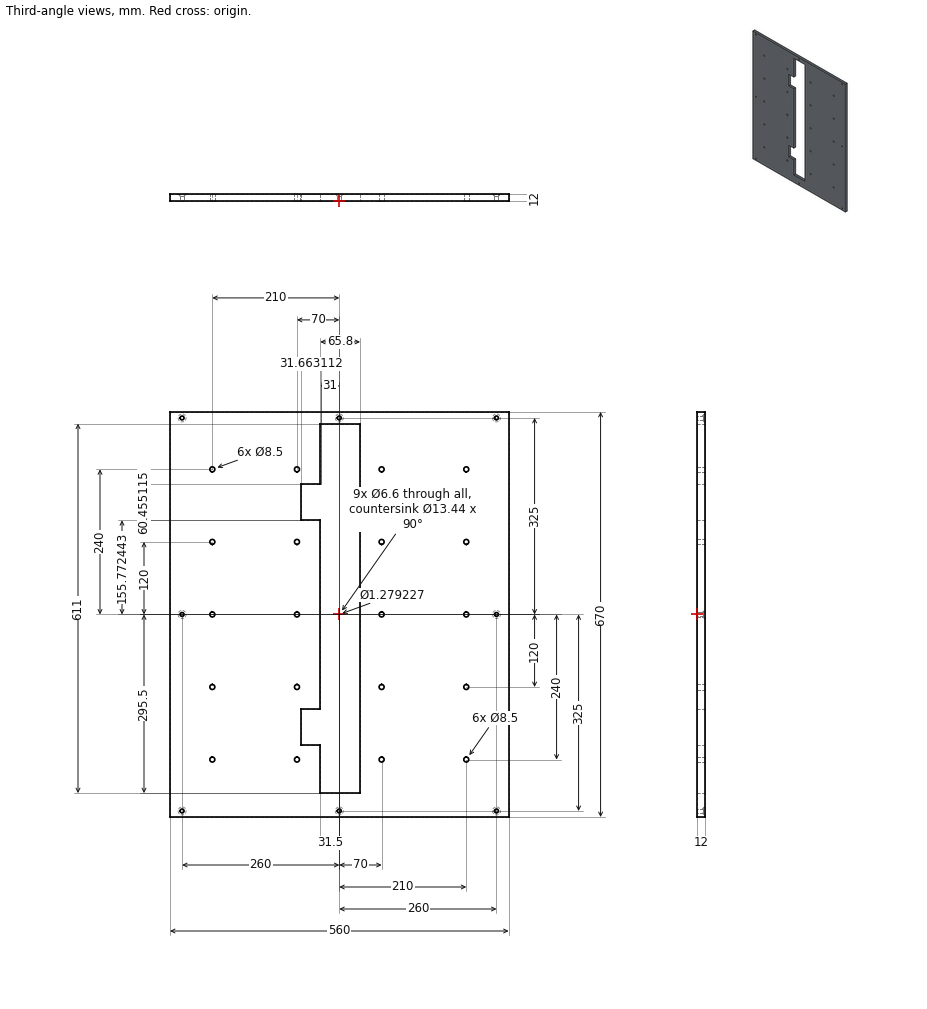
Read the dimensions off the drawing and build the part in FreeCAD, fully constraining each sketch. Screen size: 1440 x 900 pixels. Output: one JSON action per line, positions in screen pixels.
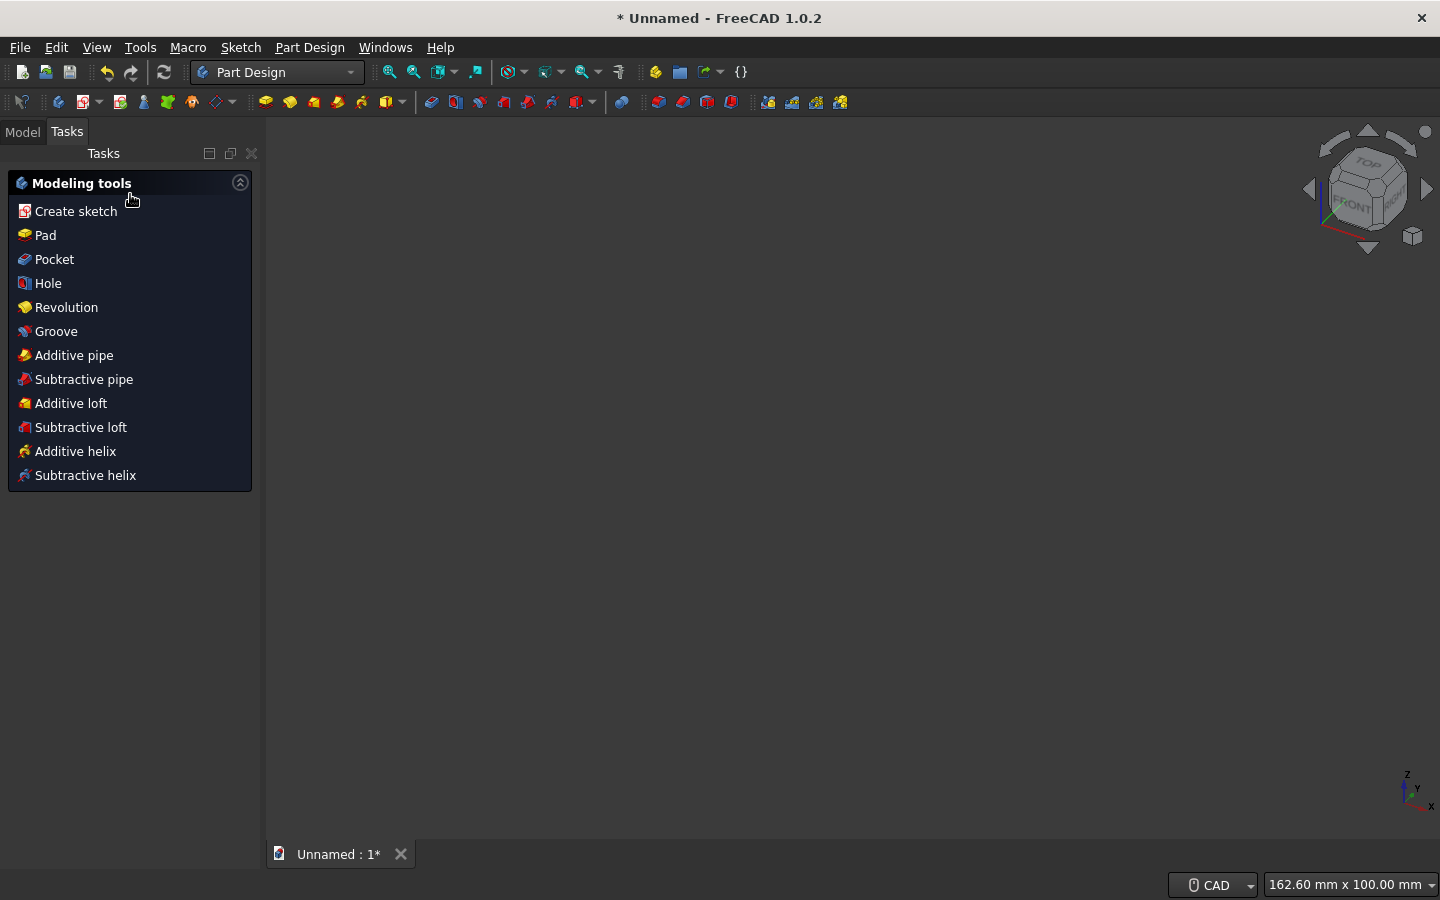
{"action": "left_click", "coordinate": [266, 102]}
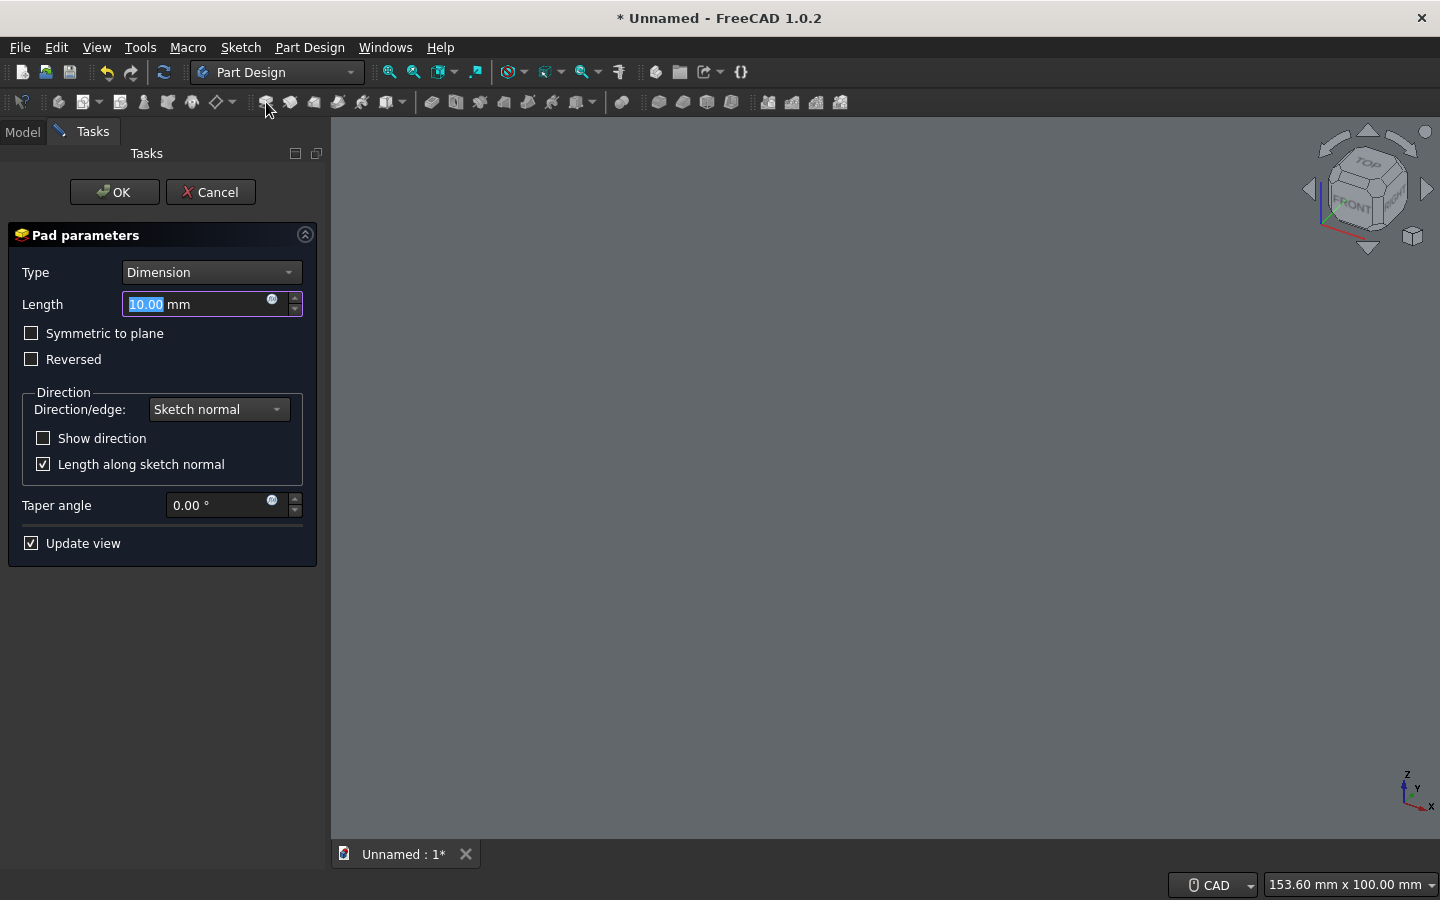
{"action": "type", "text": "12"}
{"action": "key", "text": "Tab"}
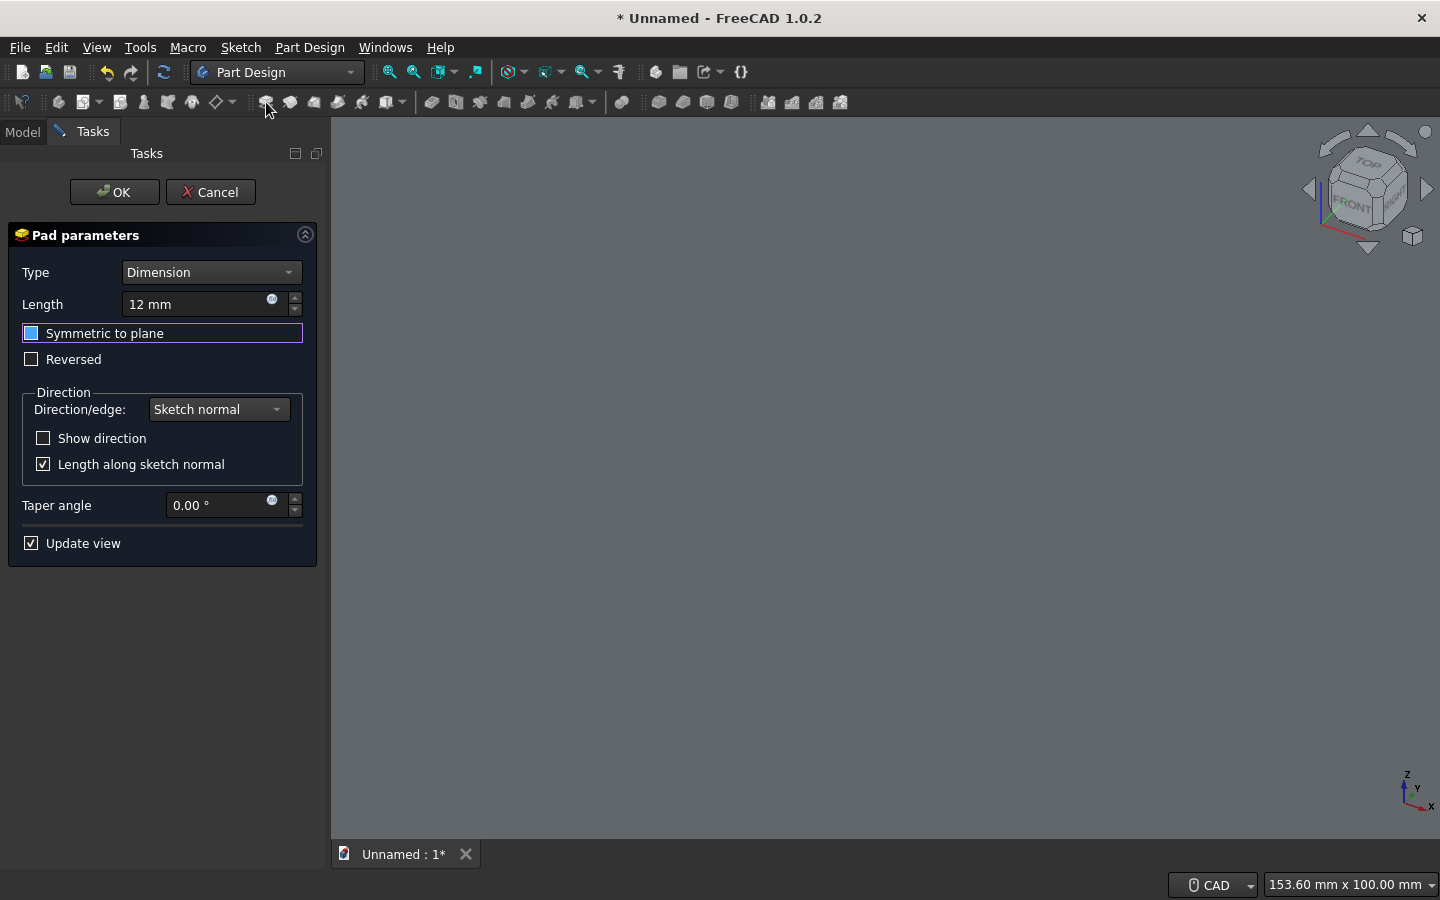
{"action": "left_click", "coordinate": [30, 359]}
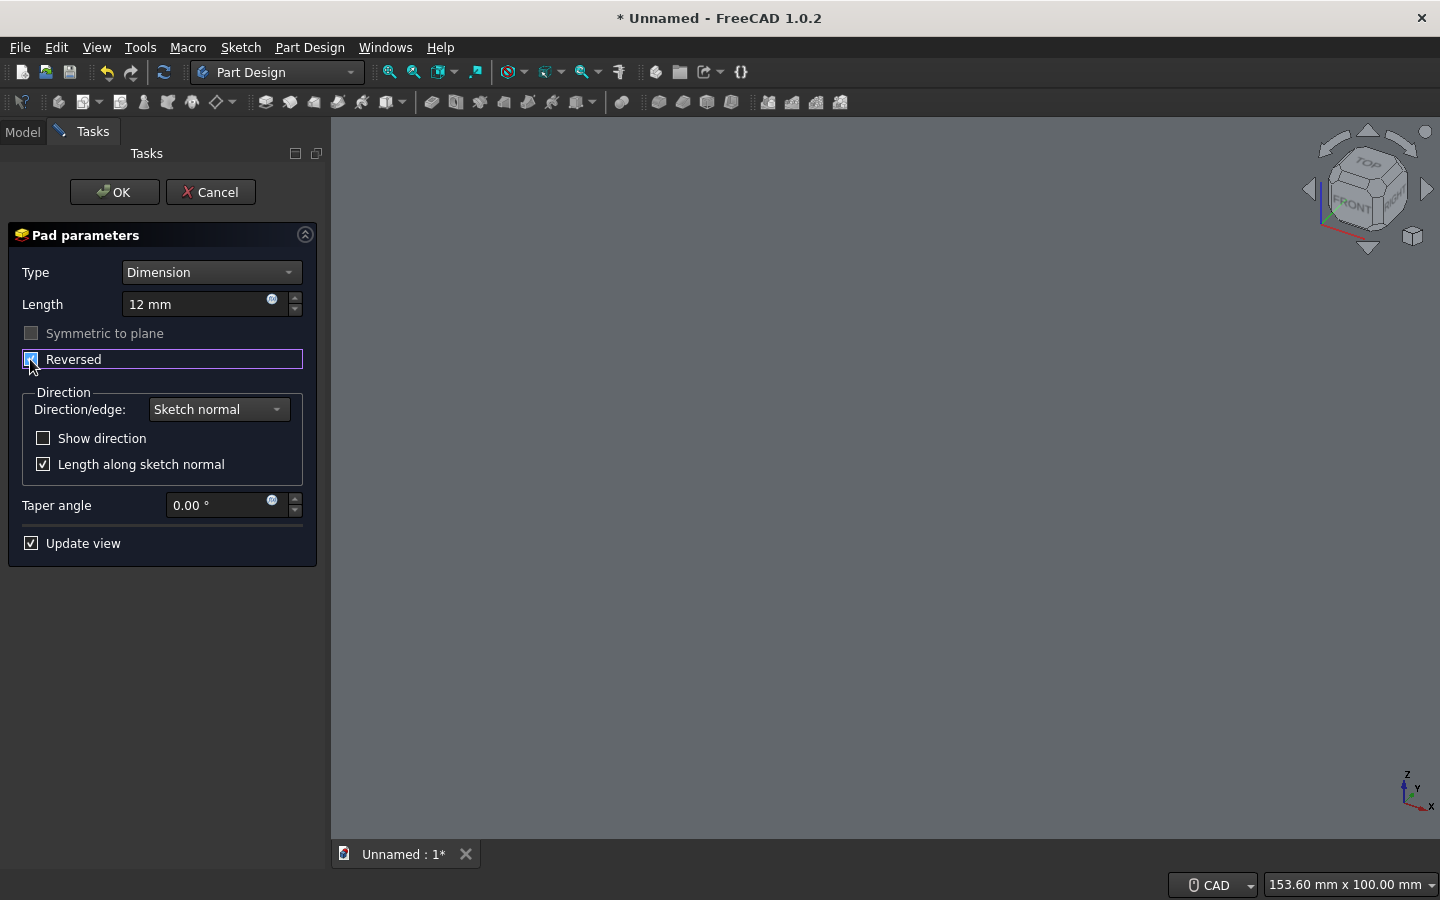
{"action": "left_click", "coordinate": [115, 192]}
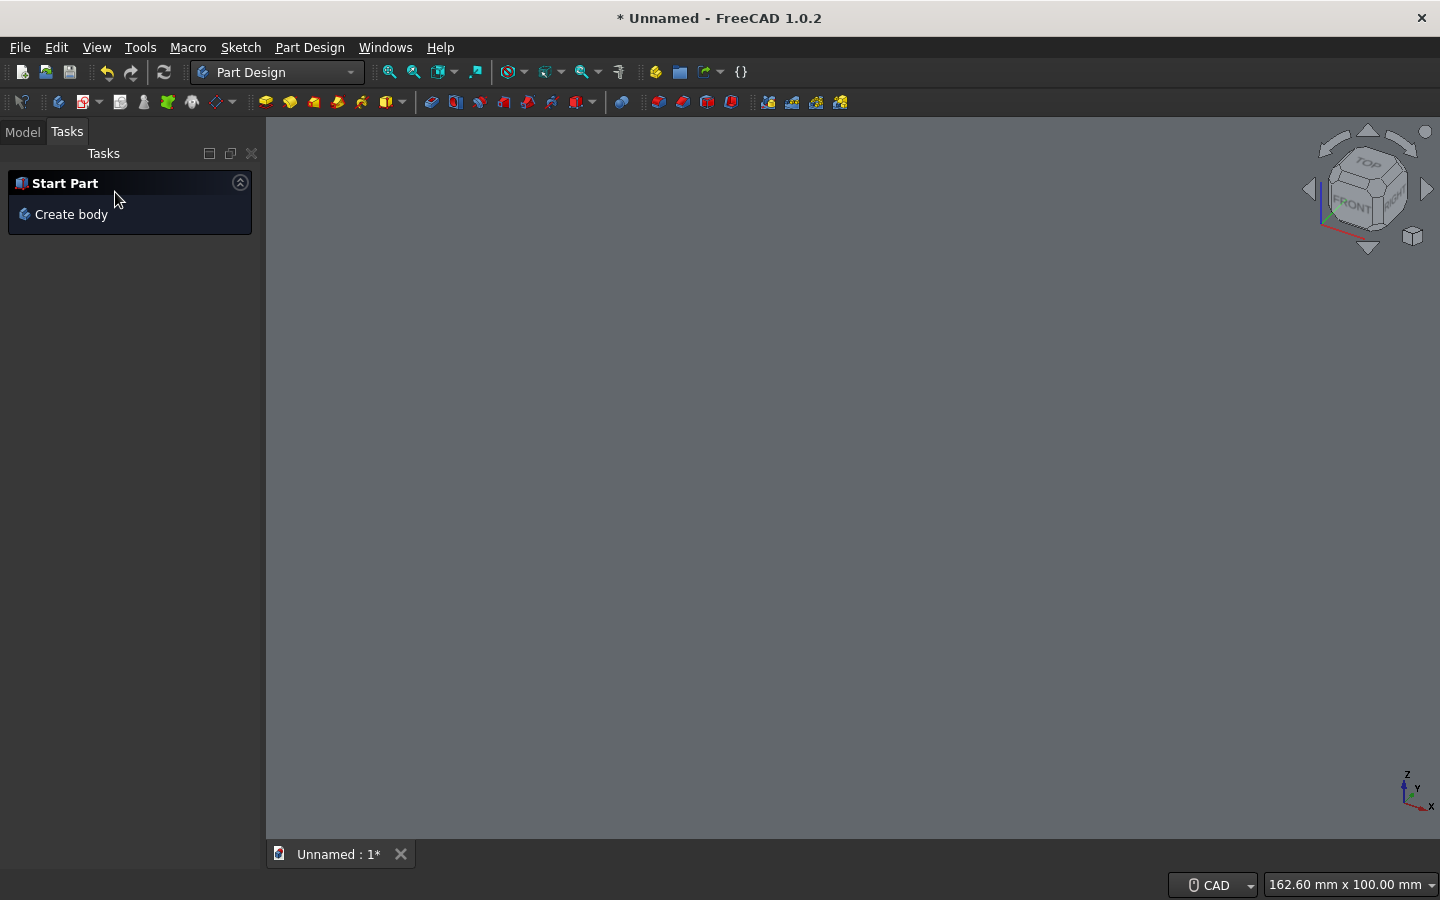
{"action": "left_click", "coordinate": [390, 72]}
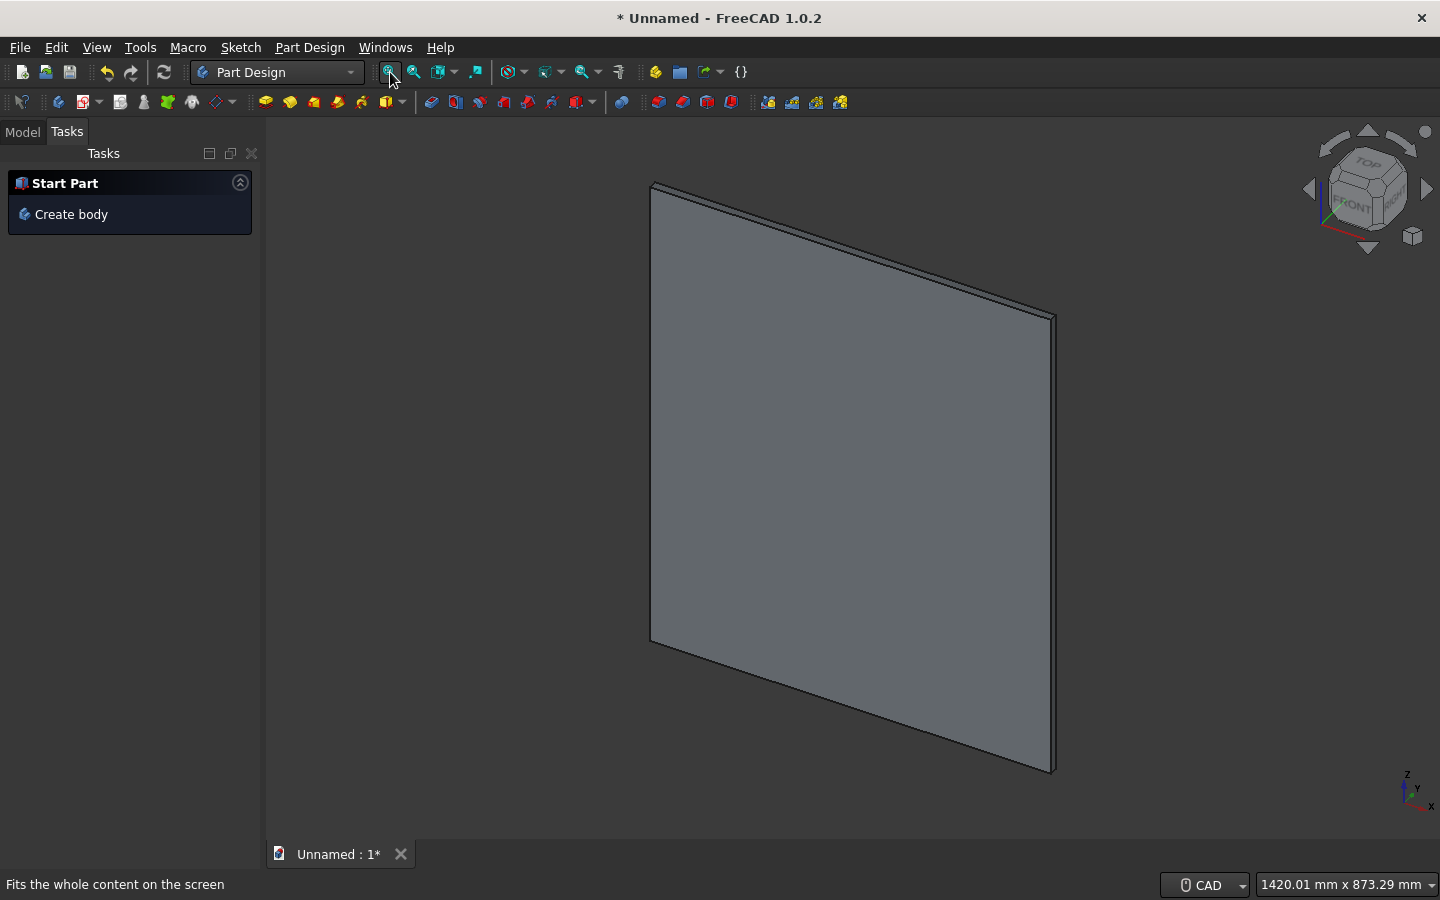
{"action": "key", "text": "4"}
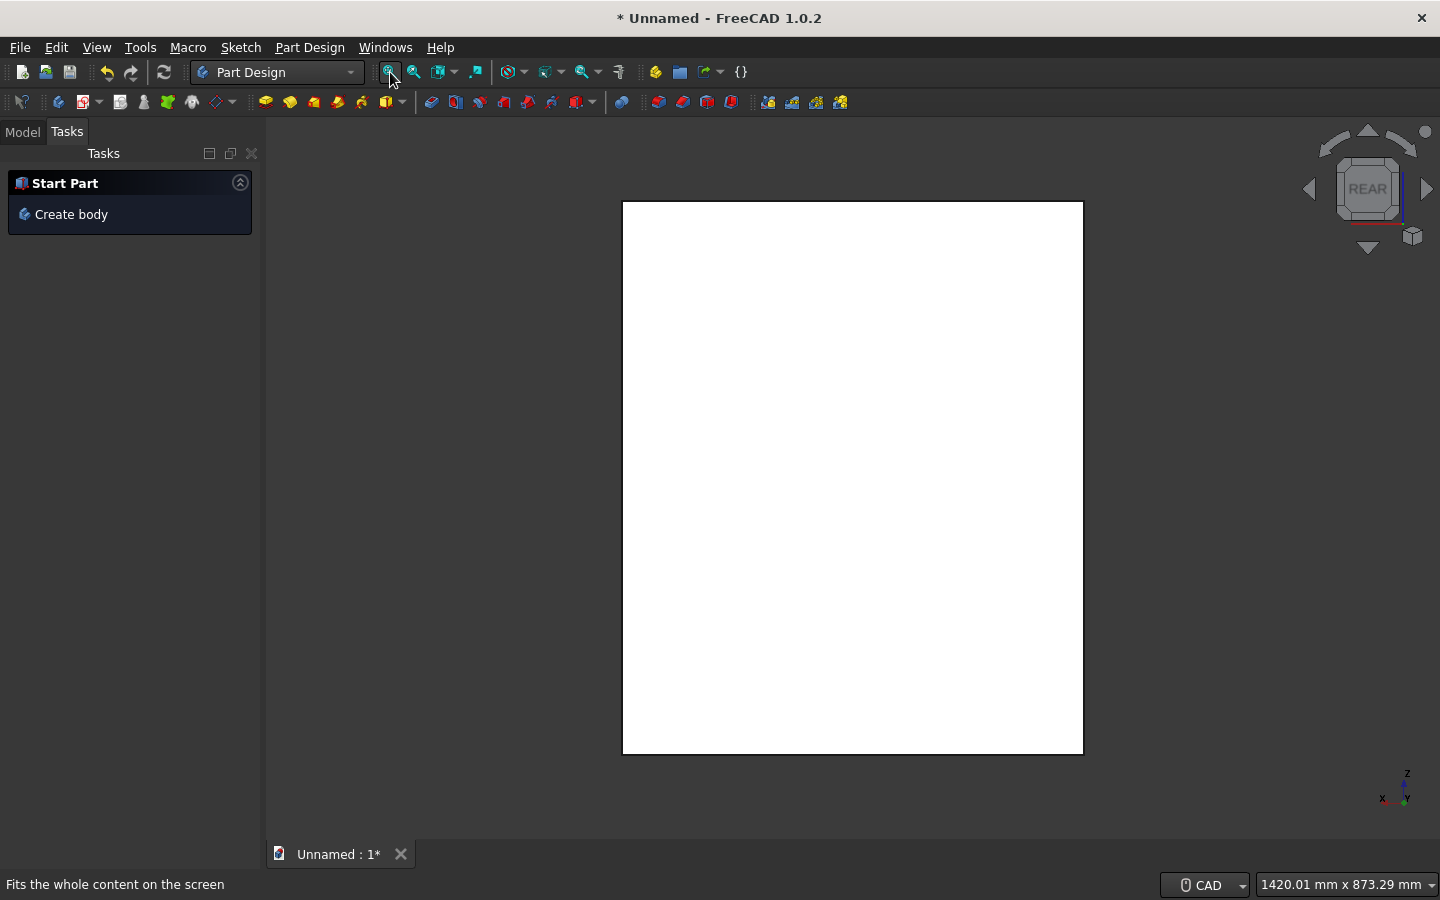
{"action": "left_click", "coordinate": [853, 477]}